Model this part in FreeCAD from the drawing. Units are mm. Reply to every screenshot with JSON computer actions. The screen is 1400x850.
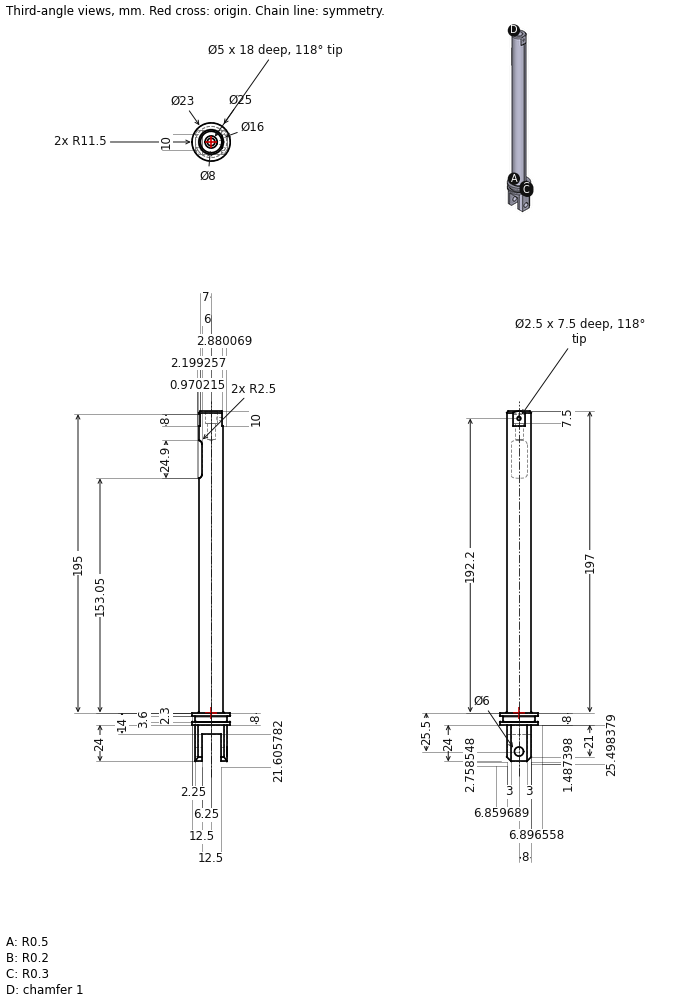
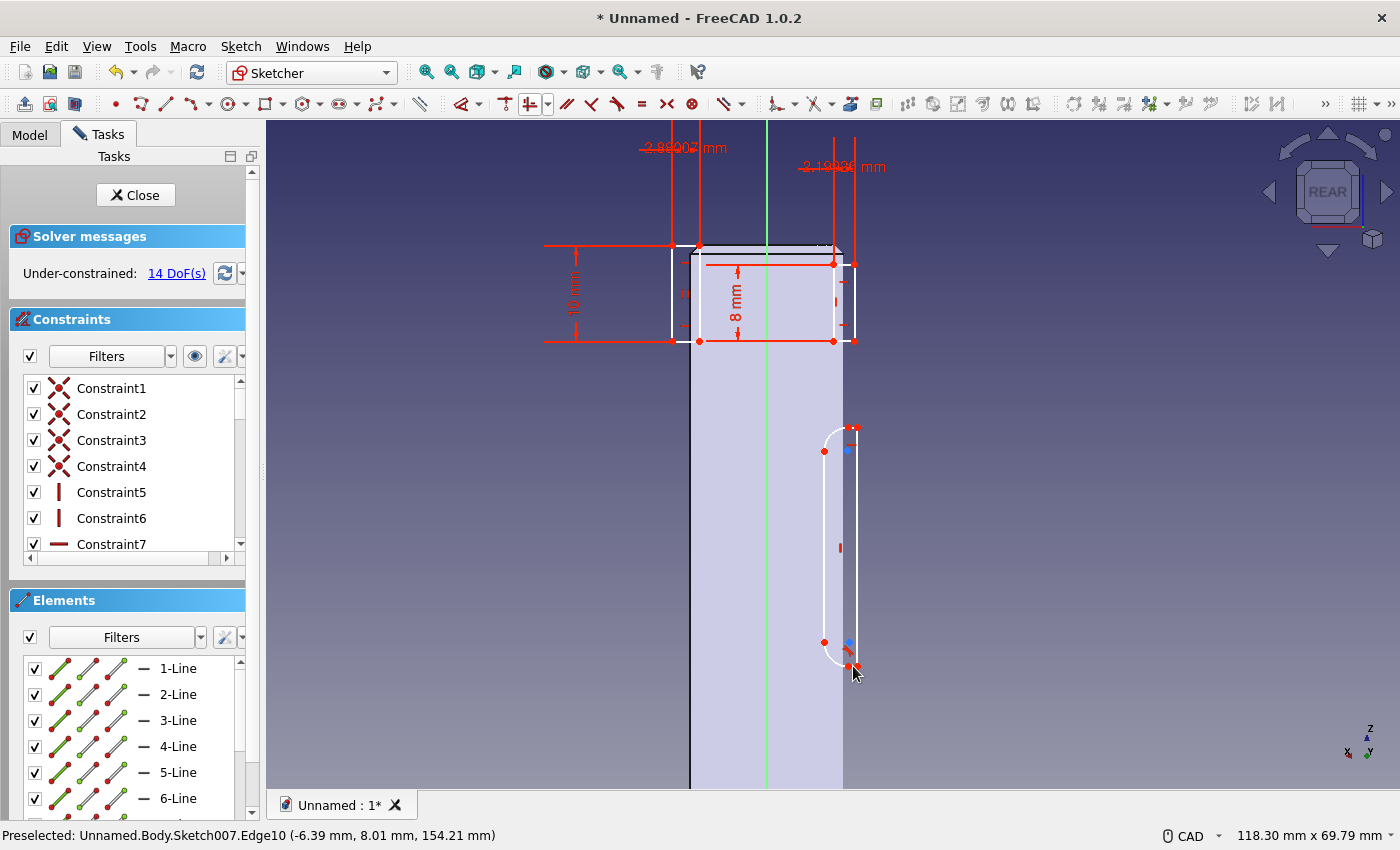
{"action": "scroll", "coordinate": [855, 428], "scroll_direction": "up", "scroll_amount": 8}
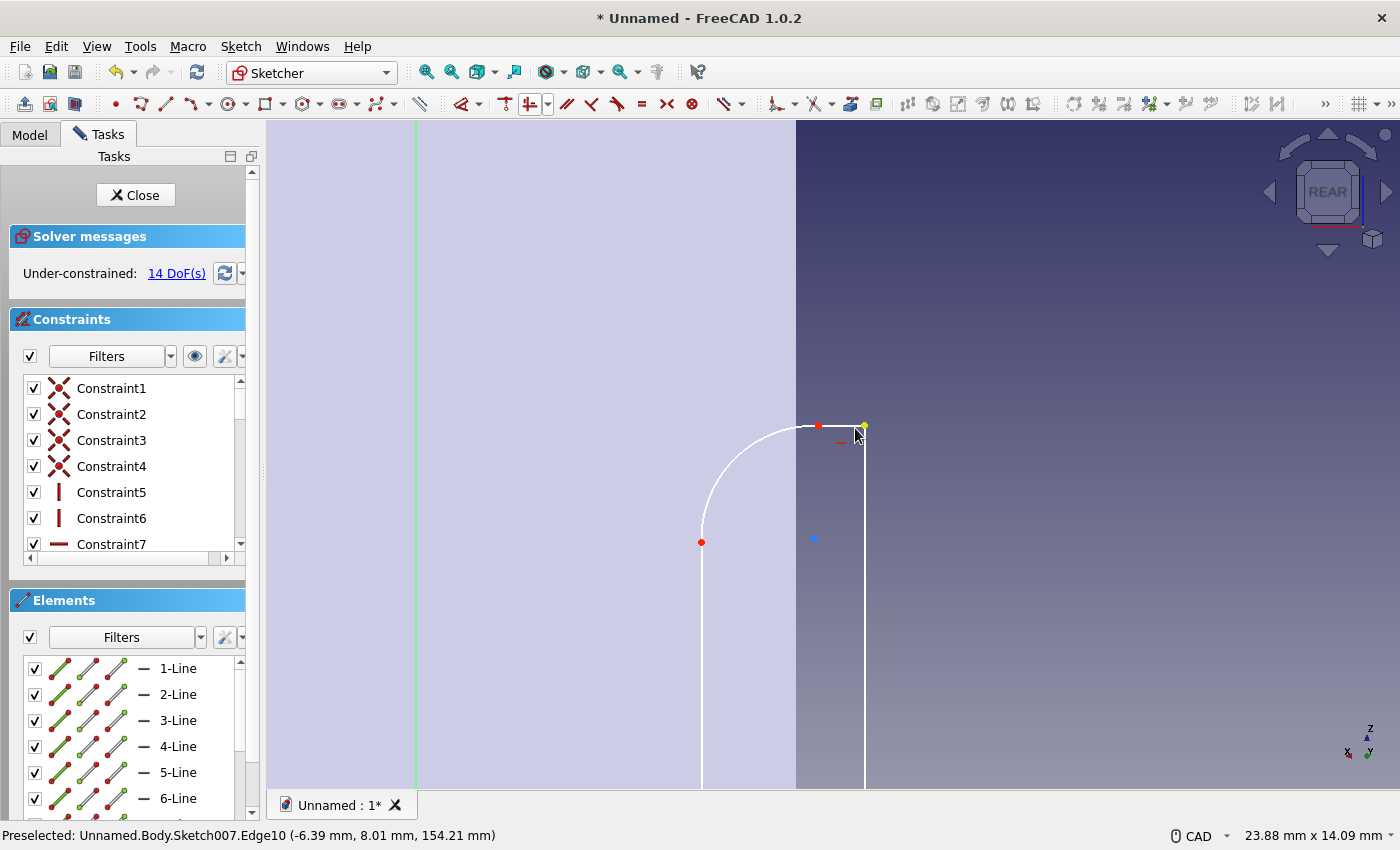
{"action": "left_click", "coordinate": [851, 426]}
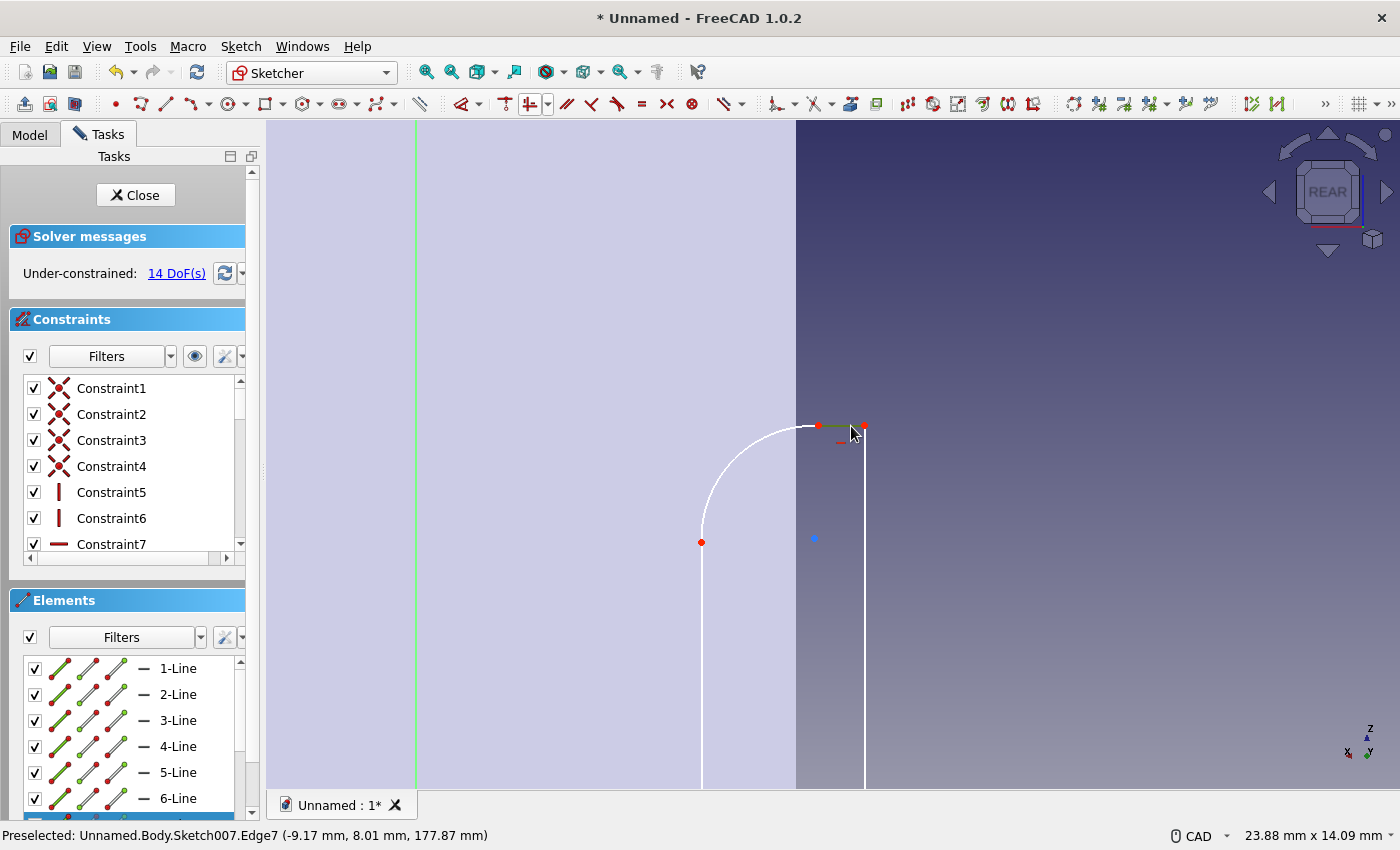
{"action": "scroll", "coordinate": [855, 428], "scroll_direction": "down", "scroll_amount": 8}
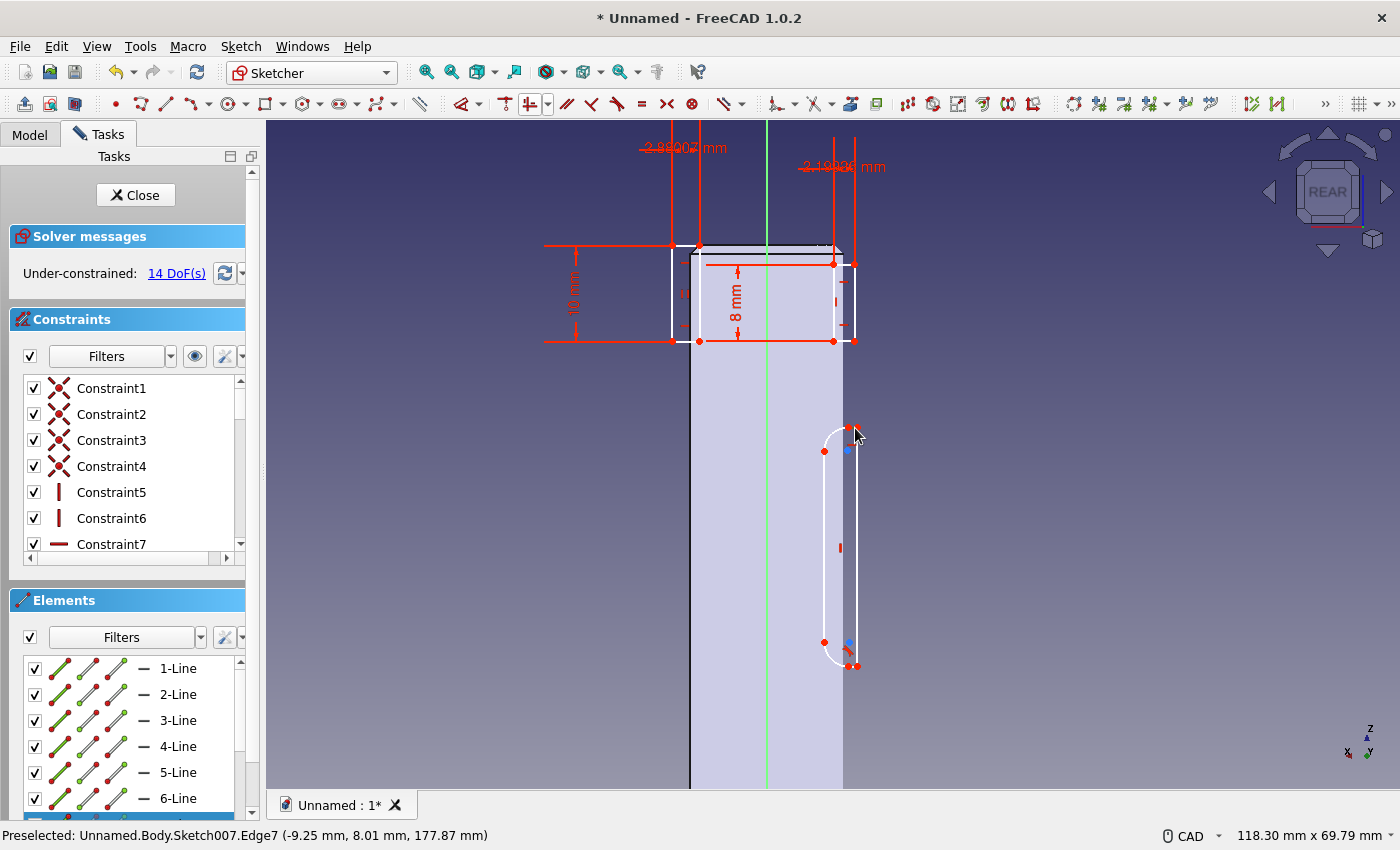
{"action": "scroll", "coordinate": [837, 430], "scroll_direction": "up", "scroll_amount": 2}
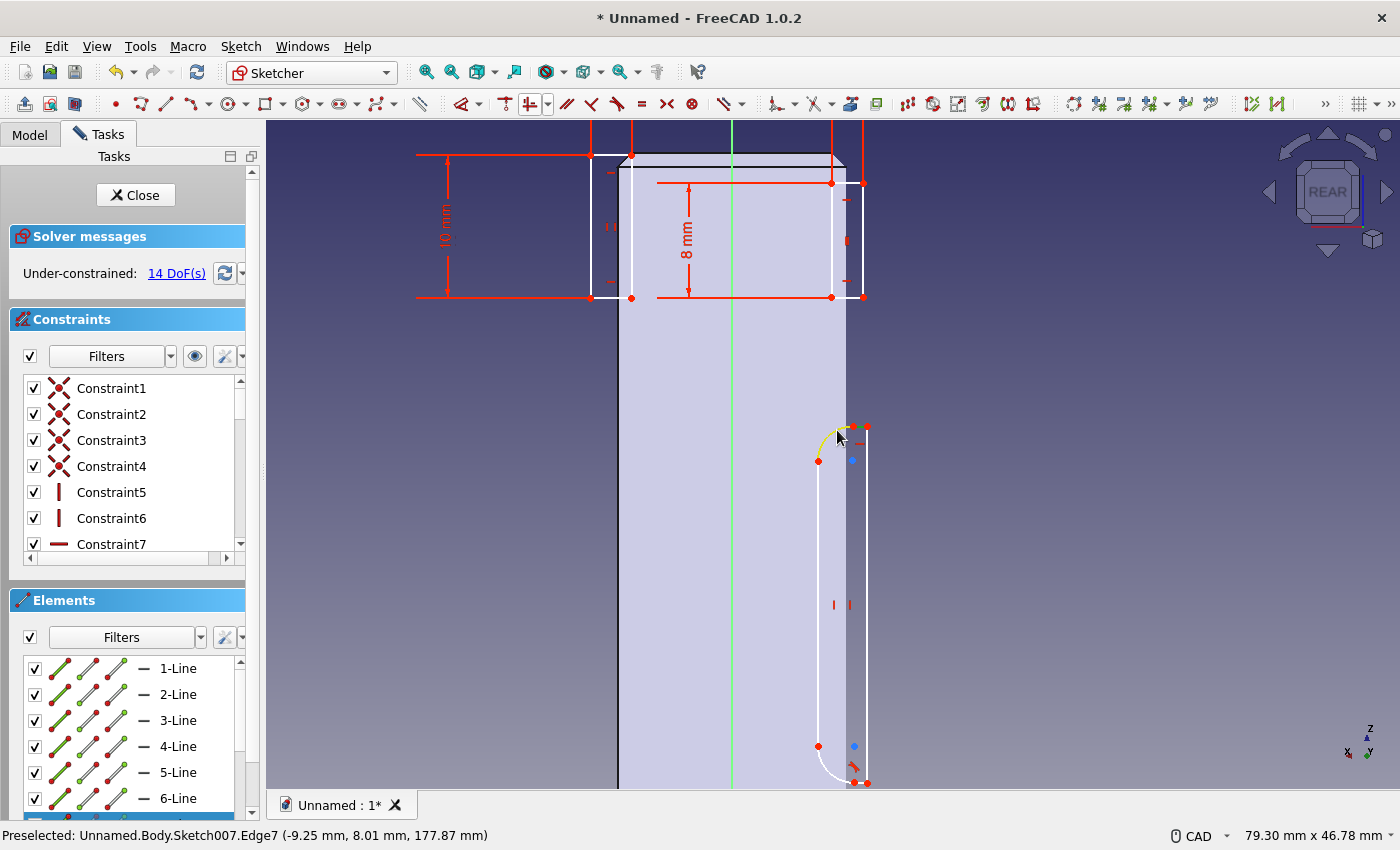
{"action": "left_click", "coordinate": [837, 430]}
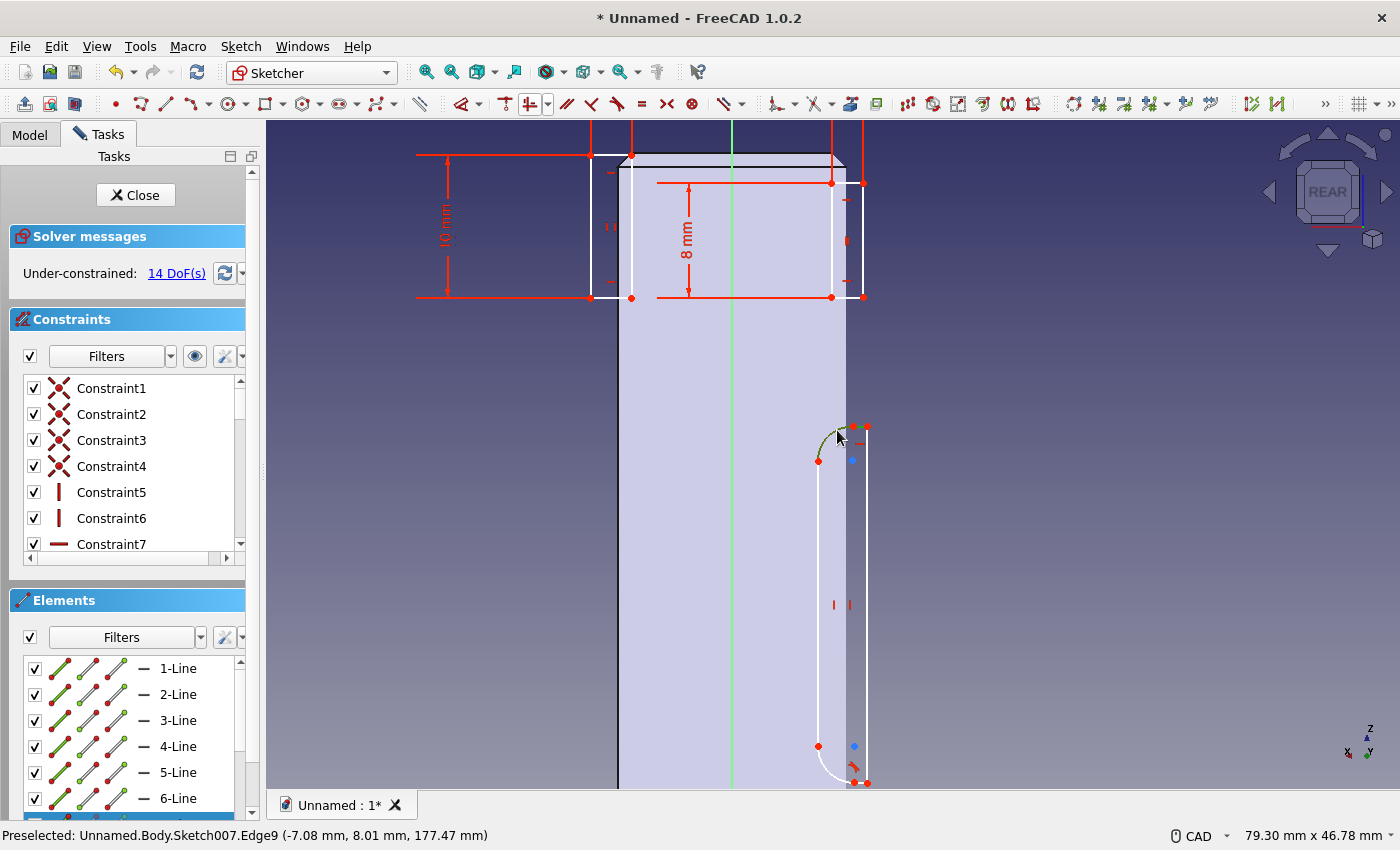
{"action": "left_click", "coordinate": [617, 104]}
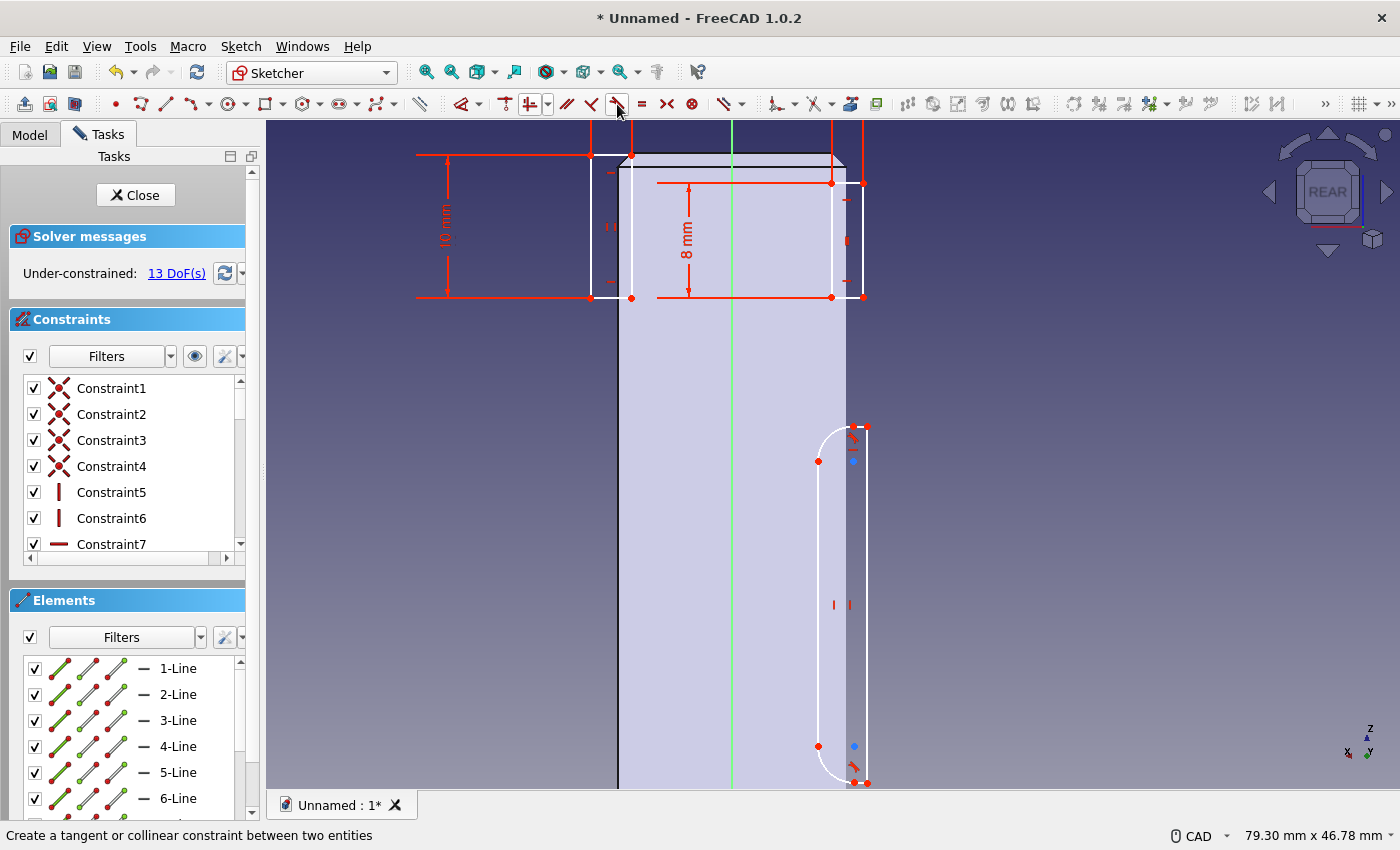
{"action": "left_click", "coordinate": [818, 547]}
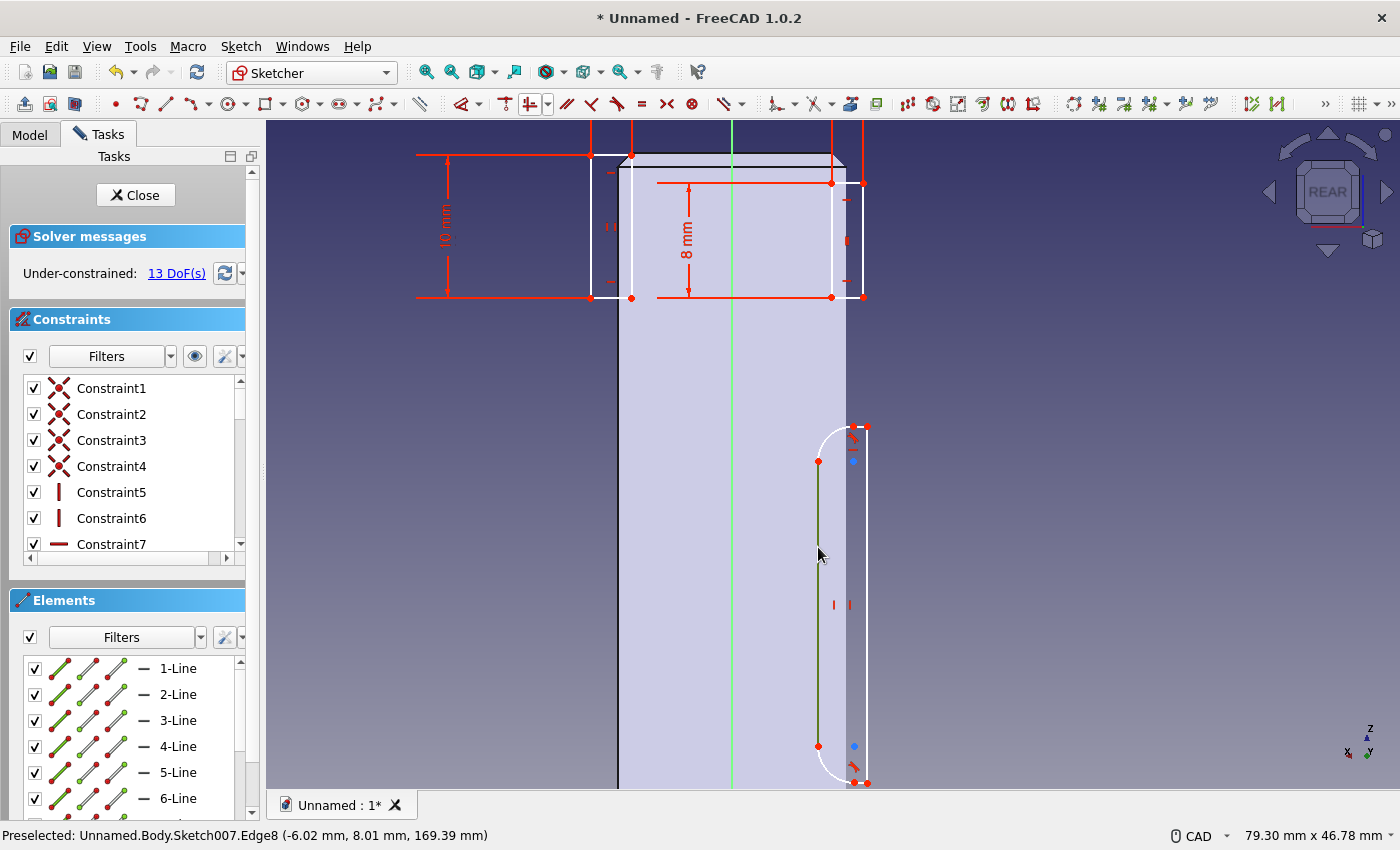
{"action": "left_click", "coordinate": [837, 431]}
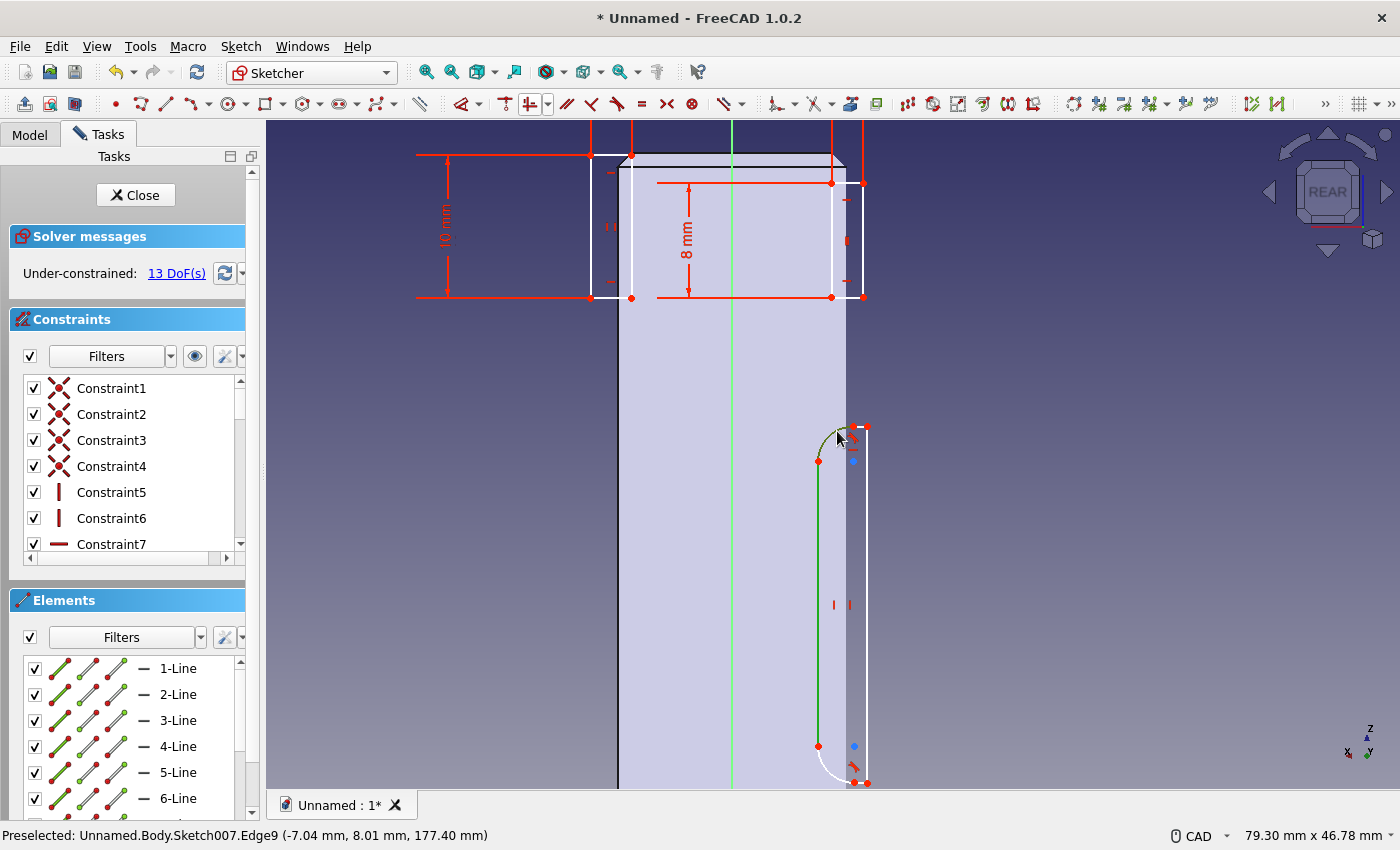
{"action": "left_click", "coordinate": [617, 104]}